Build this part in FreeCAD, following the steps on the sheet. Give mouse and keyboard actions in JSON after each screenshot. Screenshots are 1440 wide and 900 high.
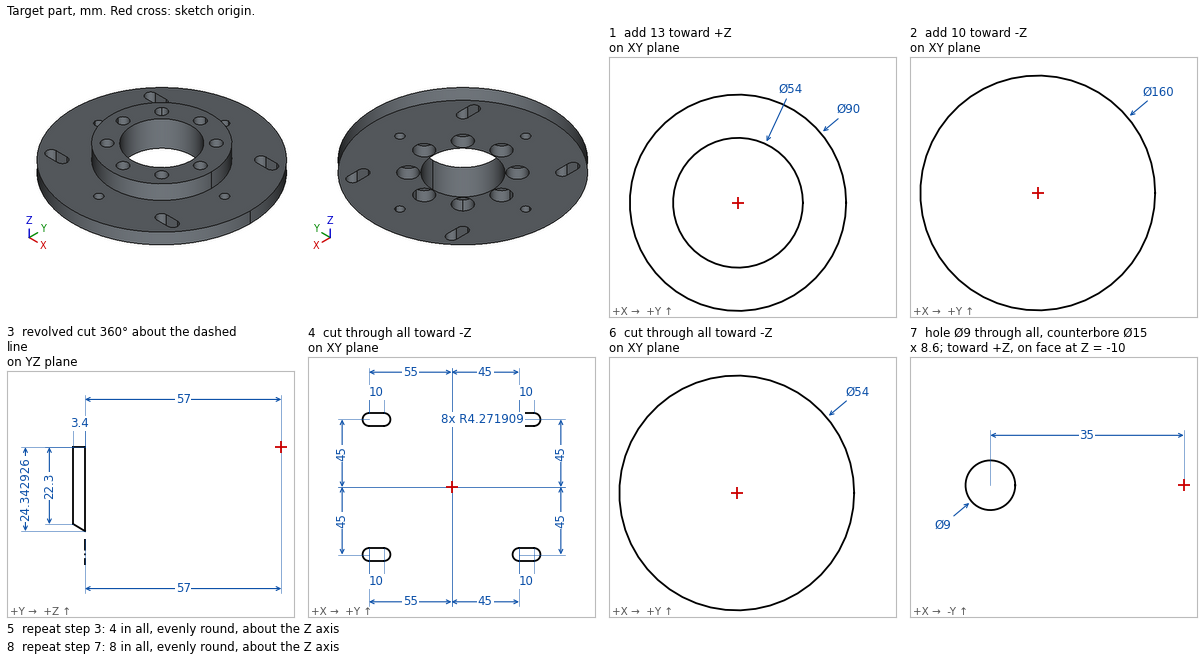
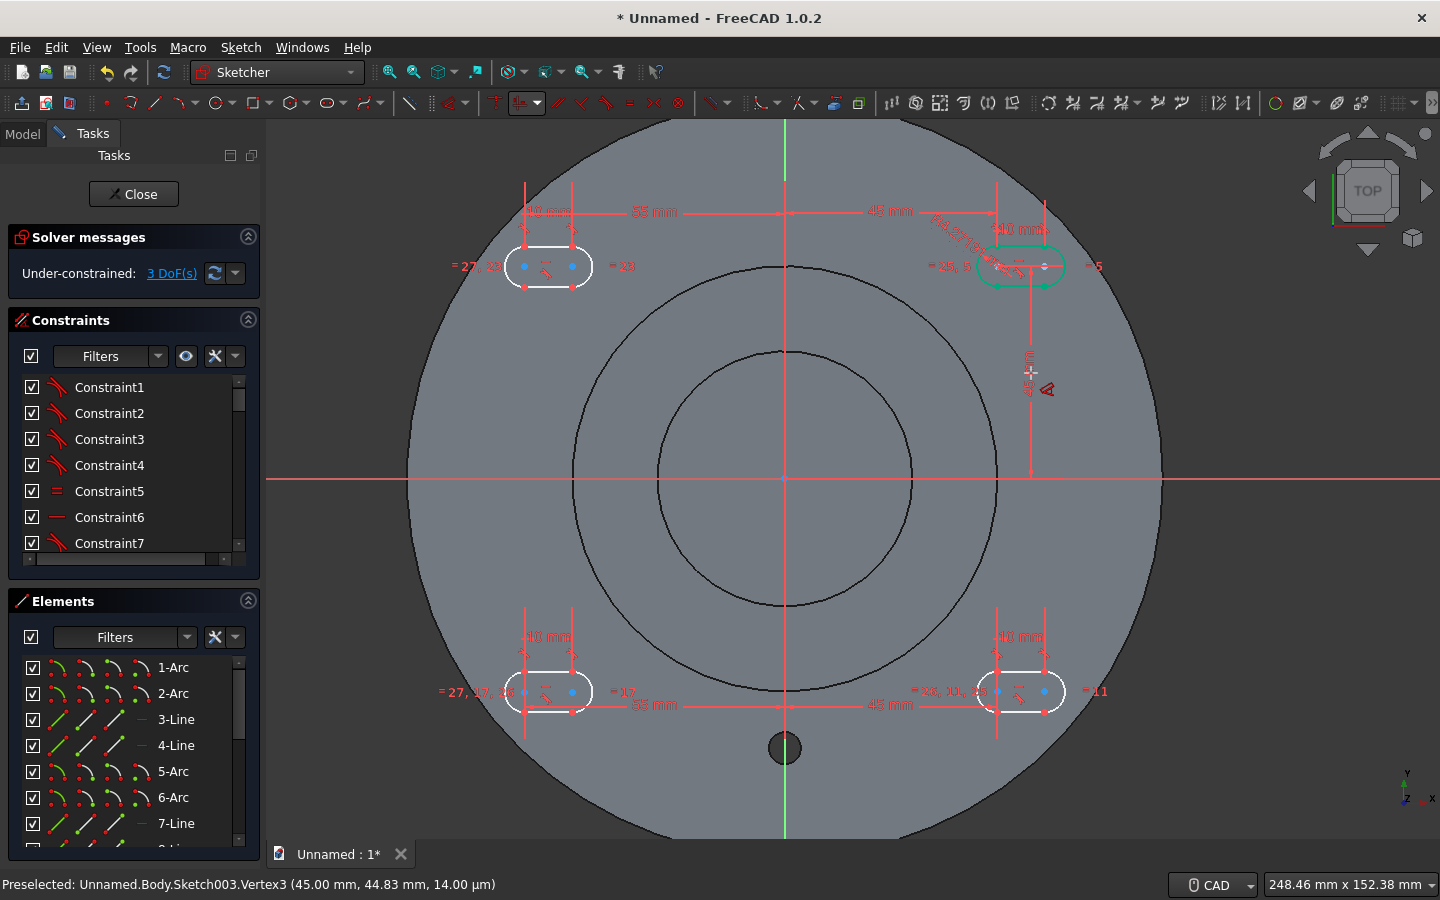
{"action": "left_click", "coordinate": [997, 692]}
{"action": "left_click", "coordinate": [1031, 585]}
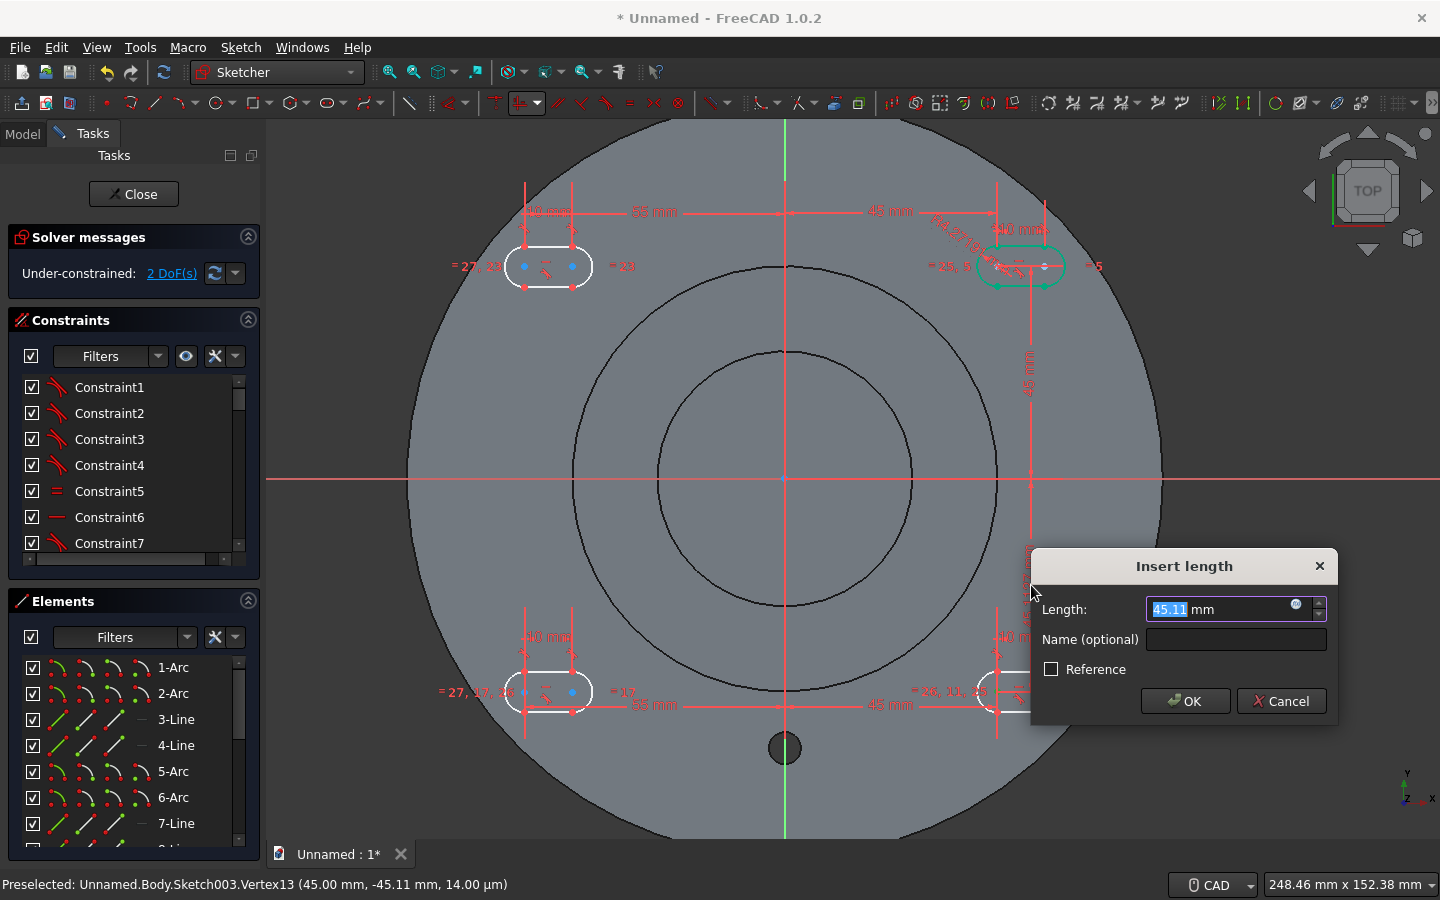
{"action": "type", "text": "45"}
{"action": "key", "text": "Return"}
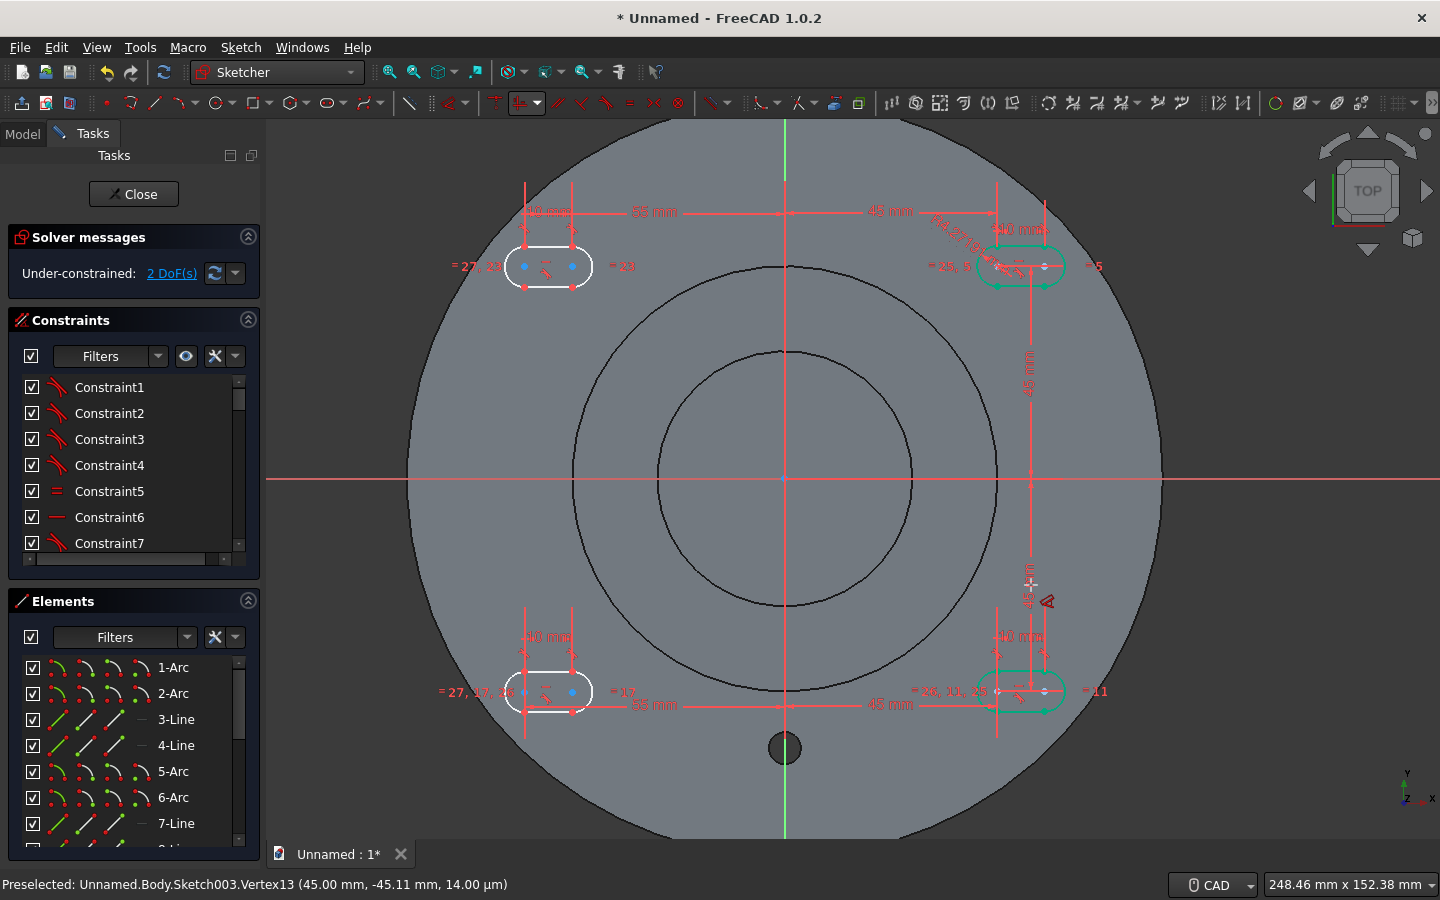
{"action": "left_click", "coordinate": [525, 692]}
{"action": "left_click", "coordinate": [491, 586]}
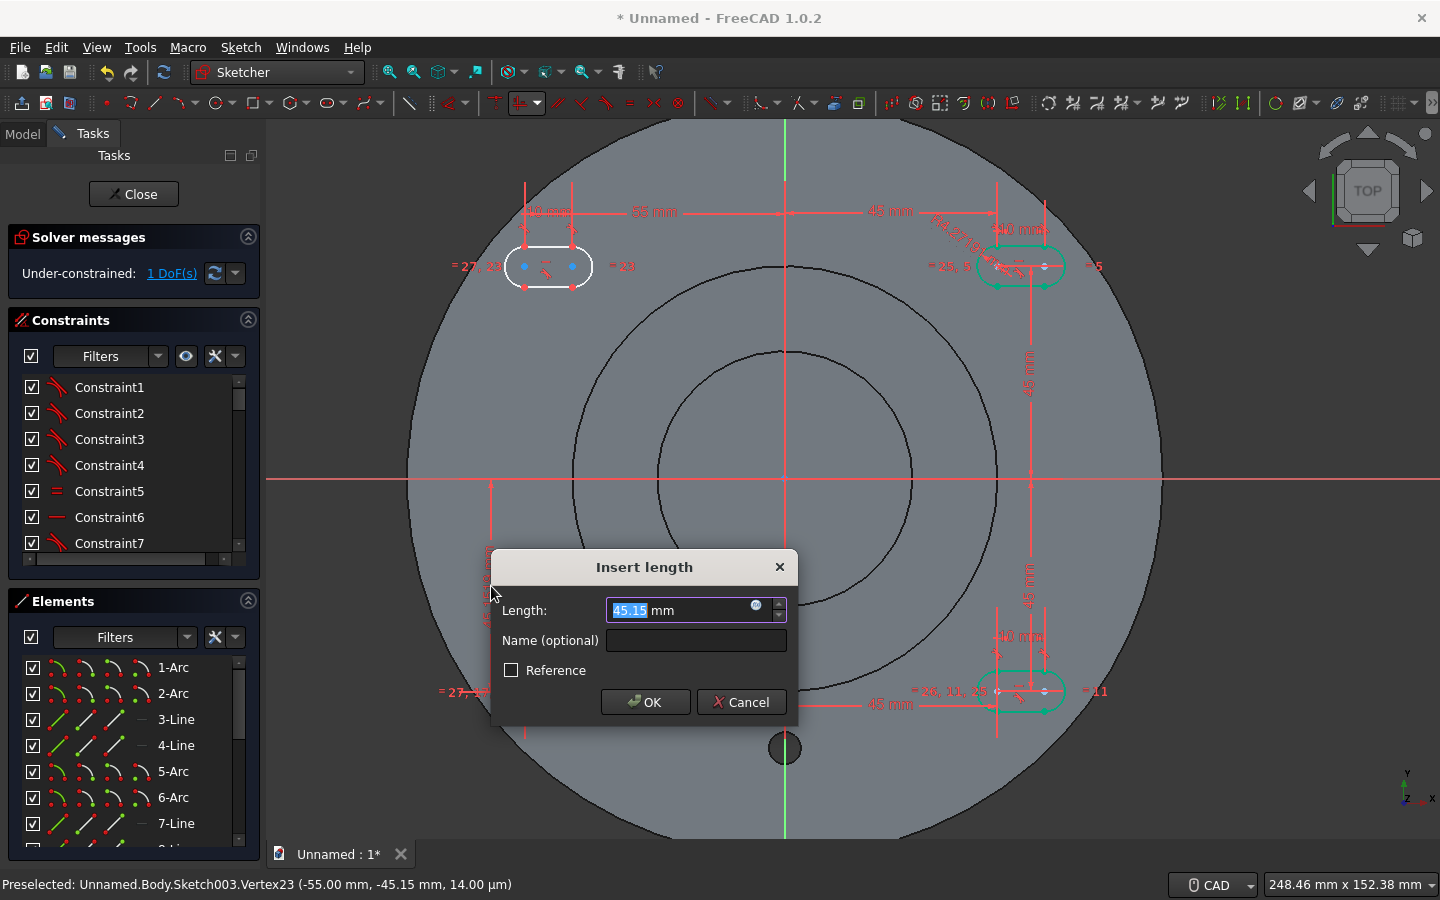
{"action": "type", "text": "45"}
{"action": "key", "text": "Return"}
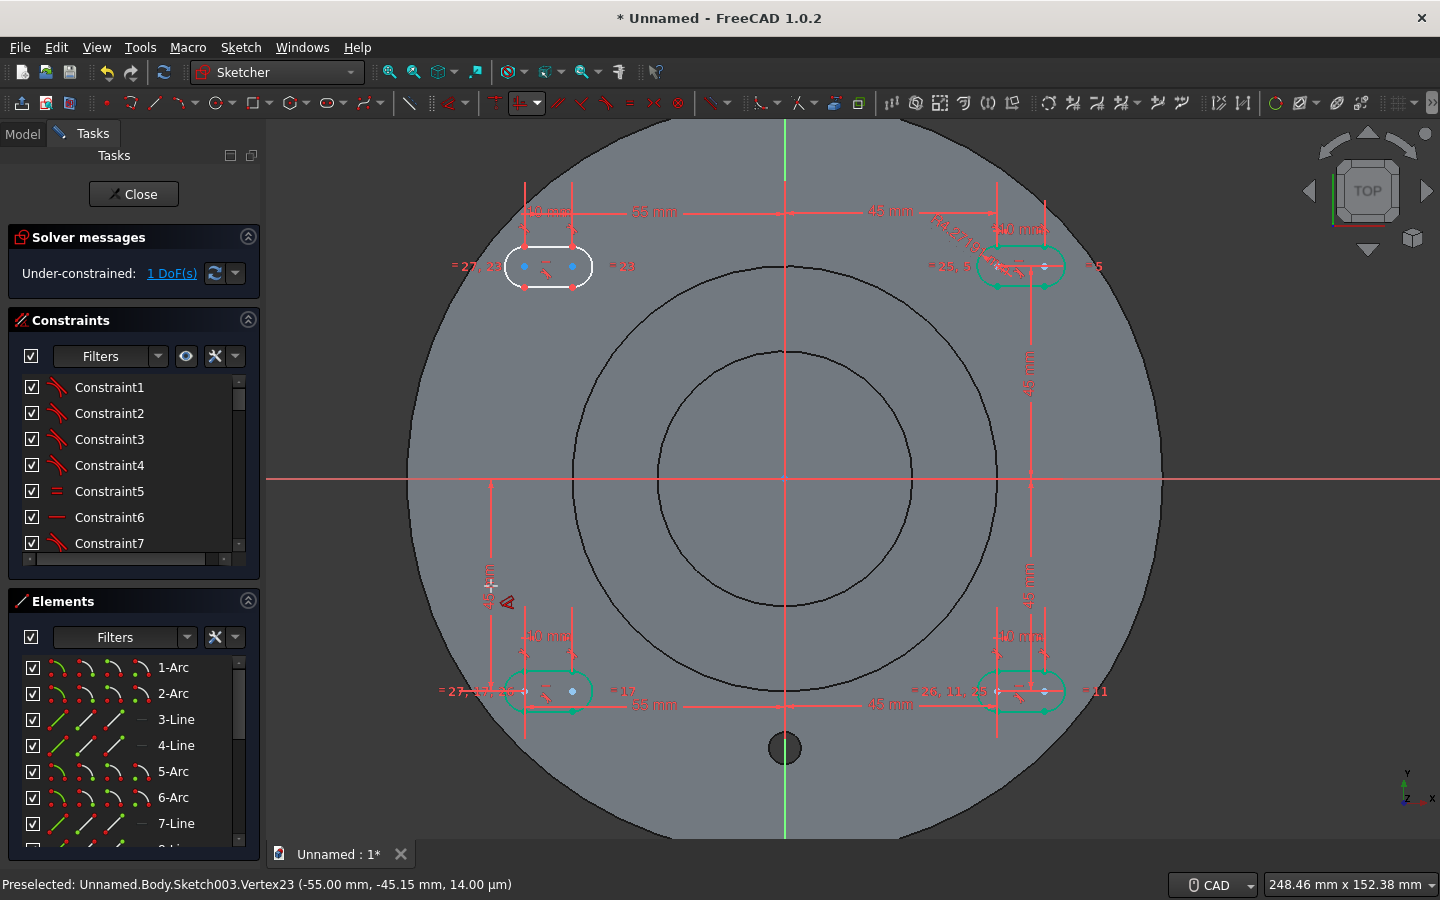
{"action": "left_click", "coordinate": [525, 267]}
{"action": "left_click", "coordinate": [491, 373]}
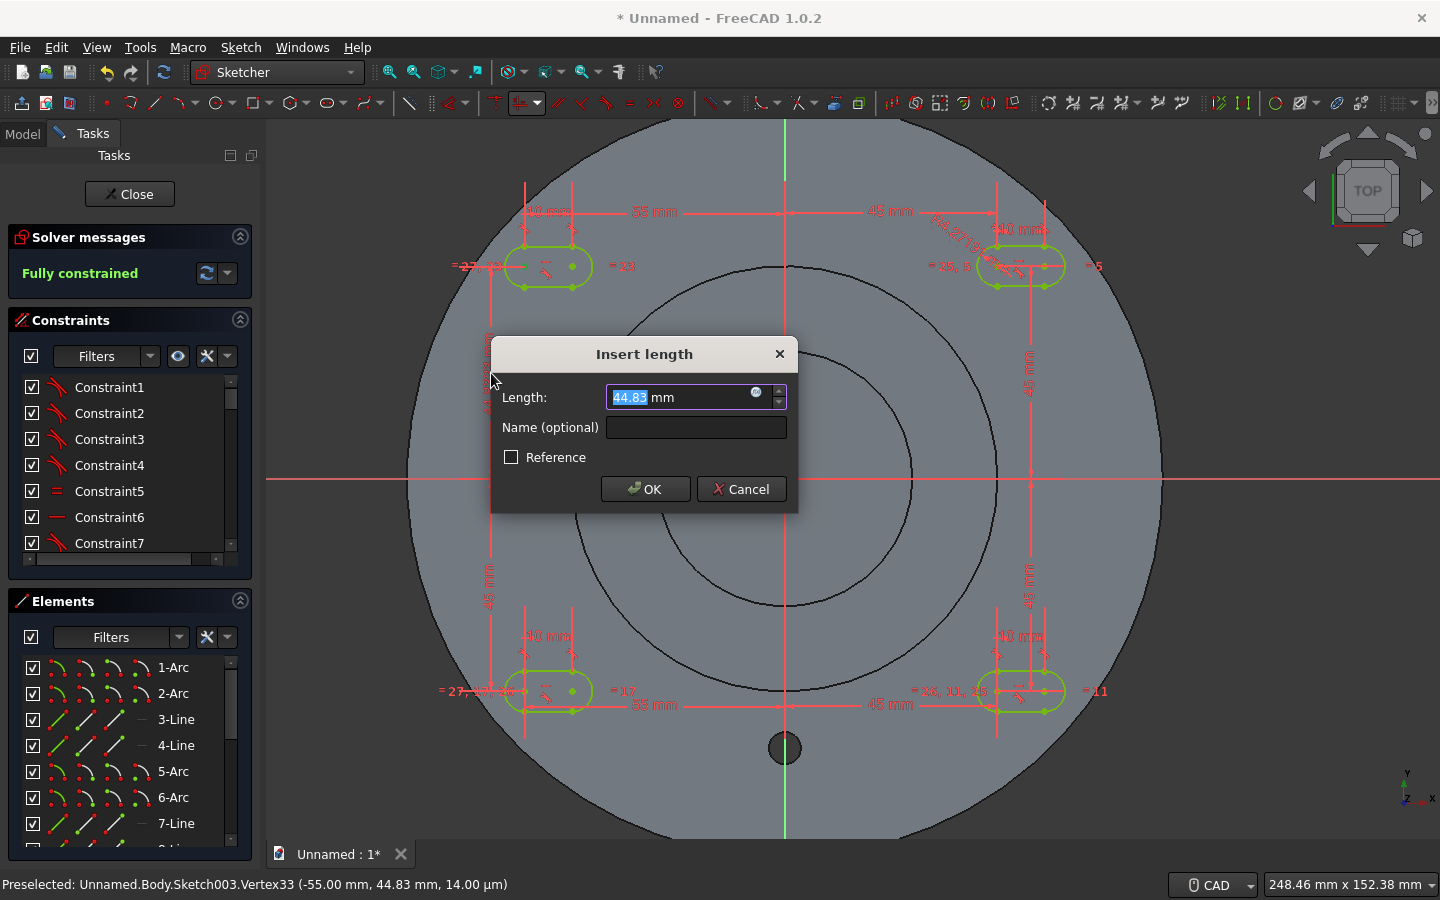
{"action": "type", "text": "45"}
{"action": "key", "text": "Return"}
{"action": "key", "text": "Escape"}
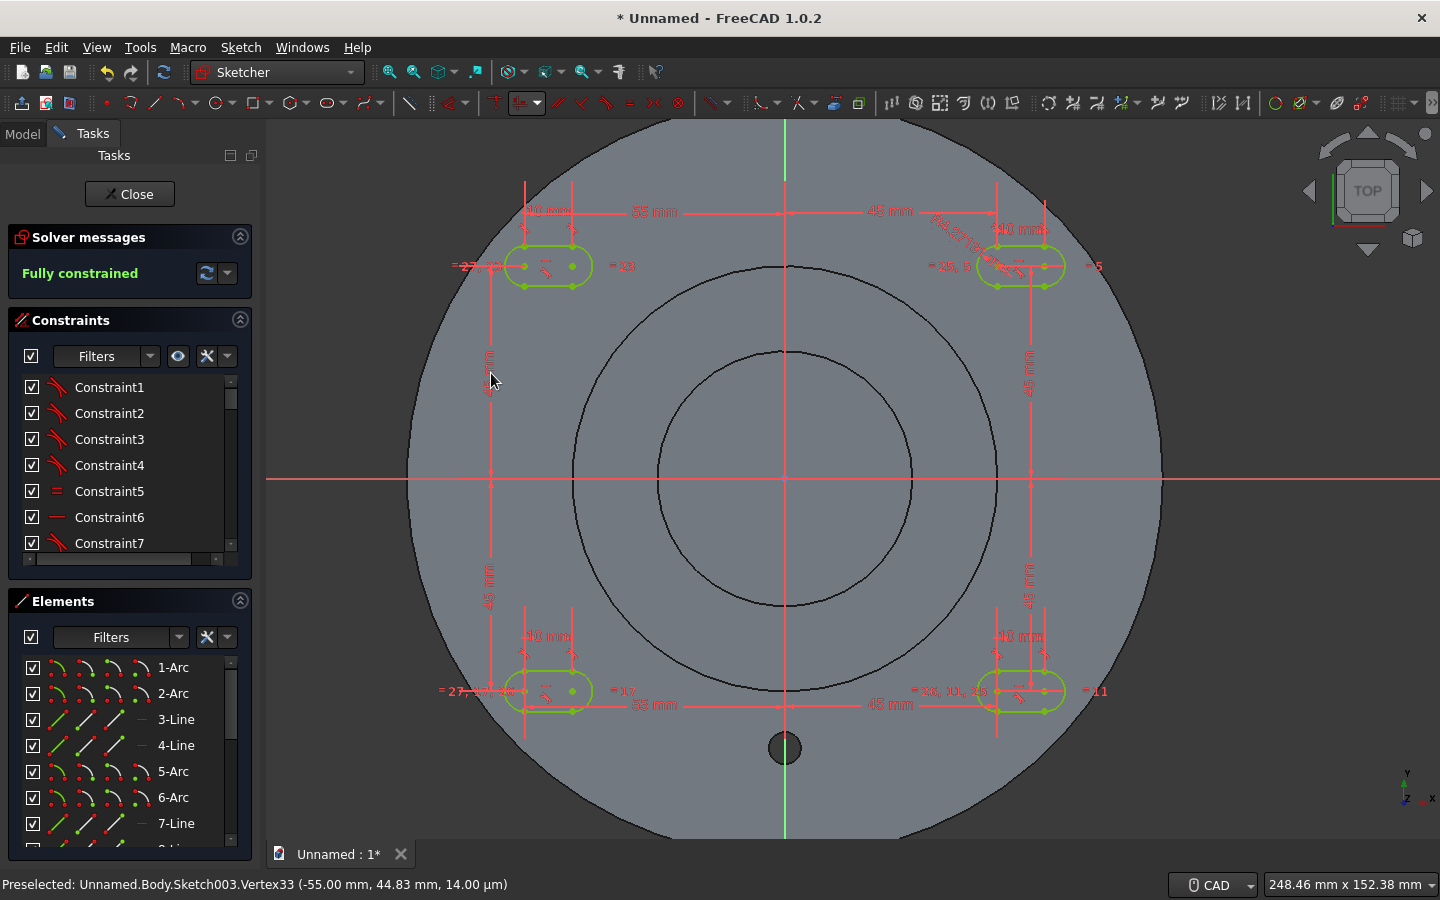
{"action": "left_click", "coordinate": [130, 194]}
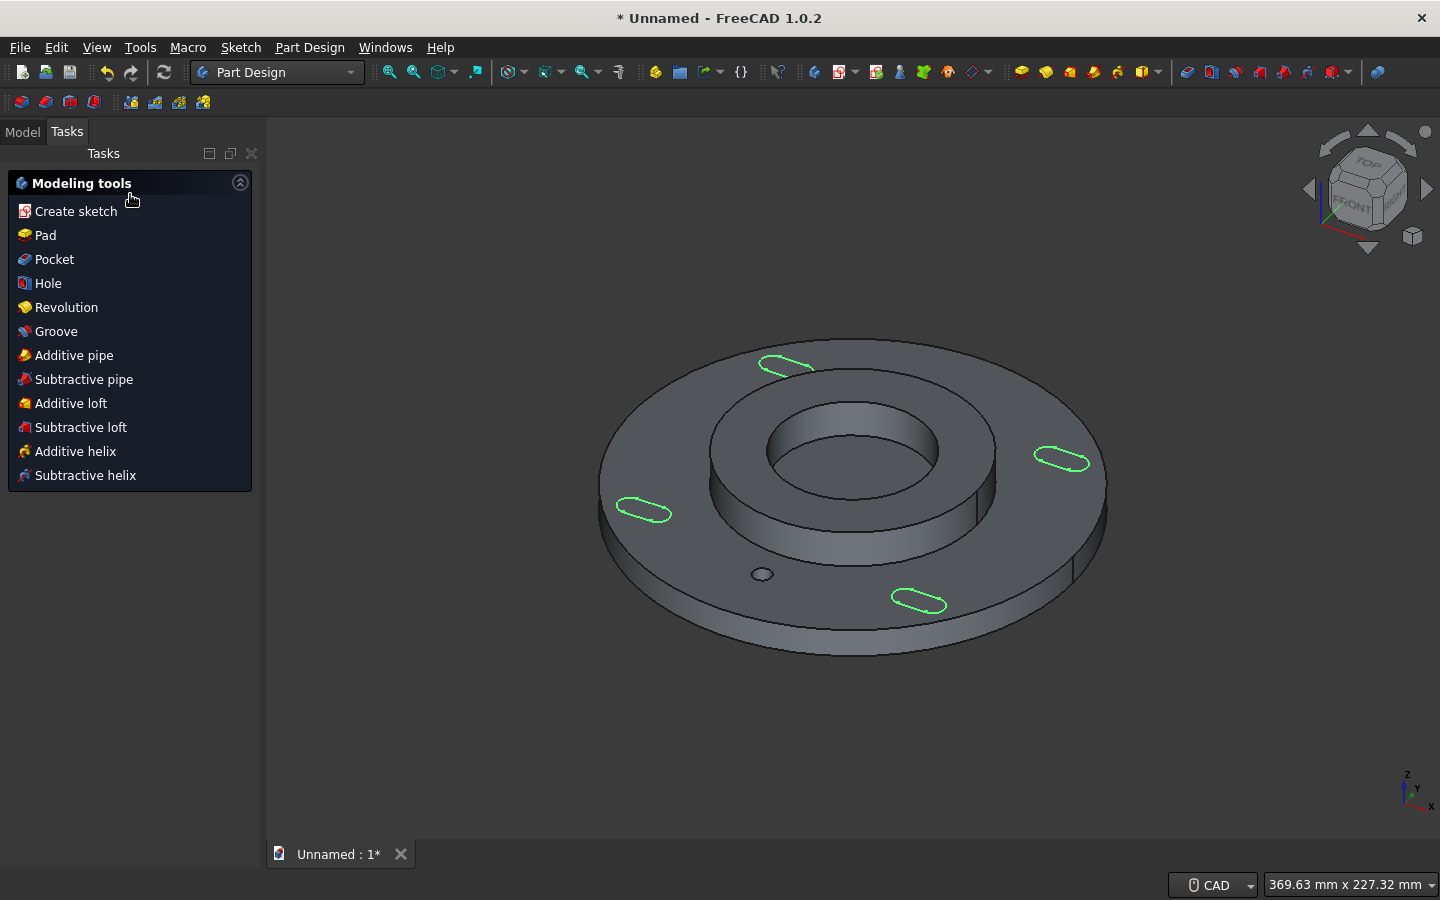
{"action": "left_click", "coordinate": [1188, 72]}